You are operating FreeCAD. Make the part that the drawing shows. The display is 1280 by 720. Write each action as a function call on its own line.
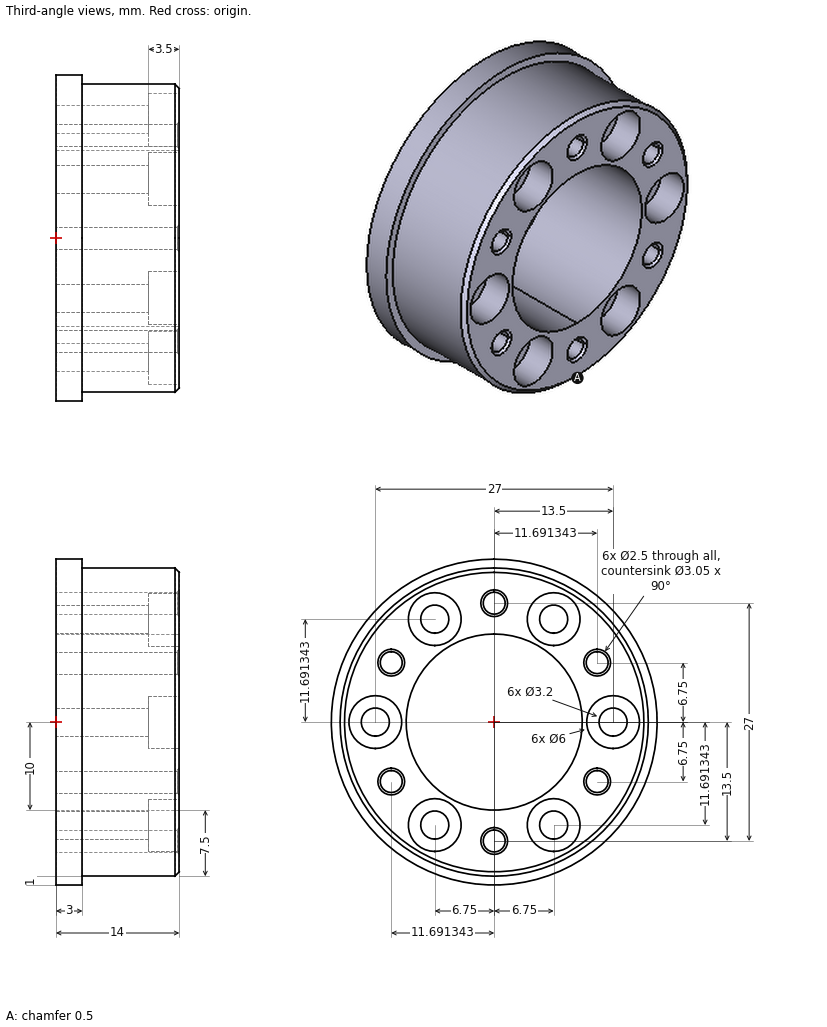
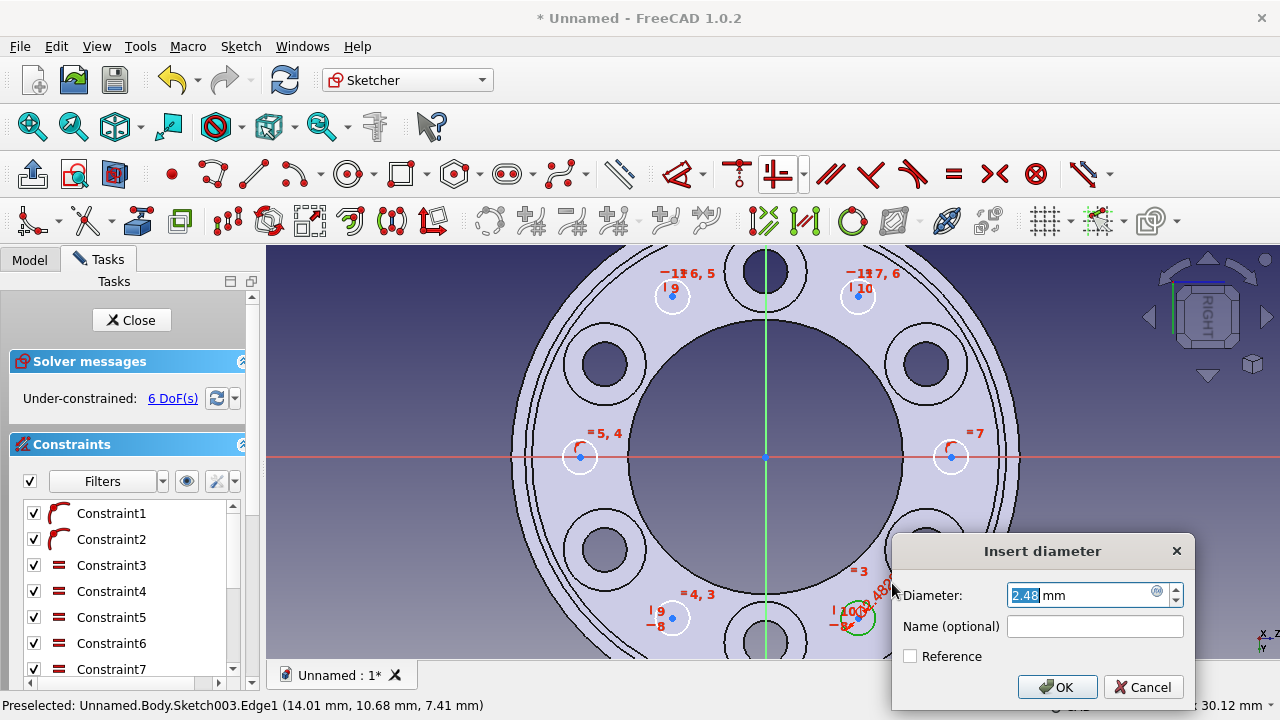
text(2.5)
key(Return)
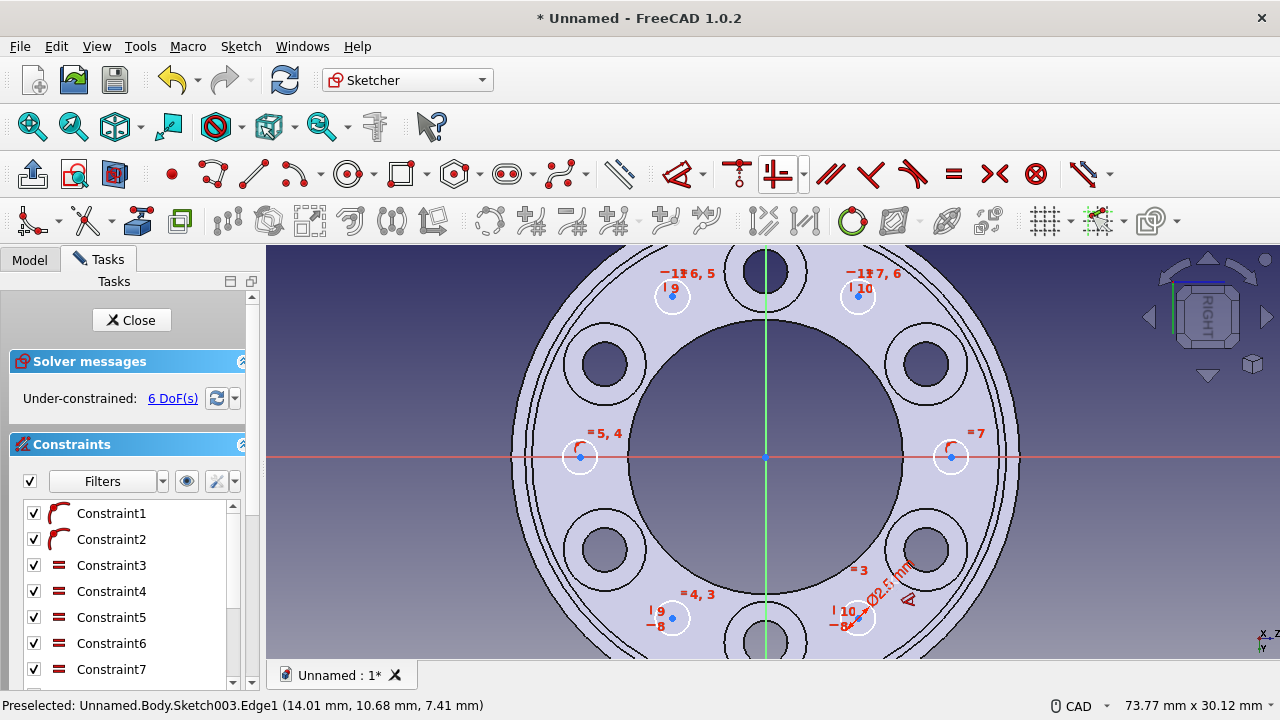
click(580, 457)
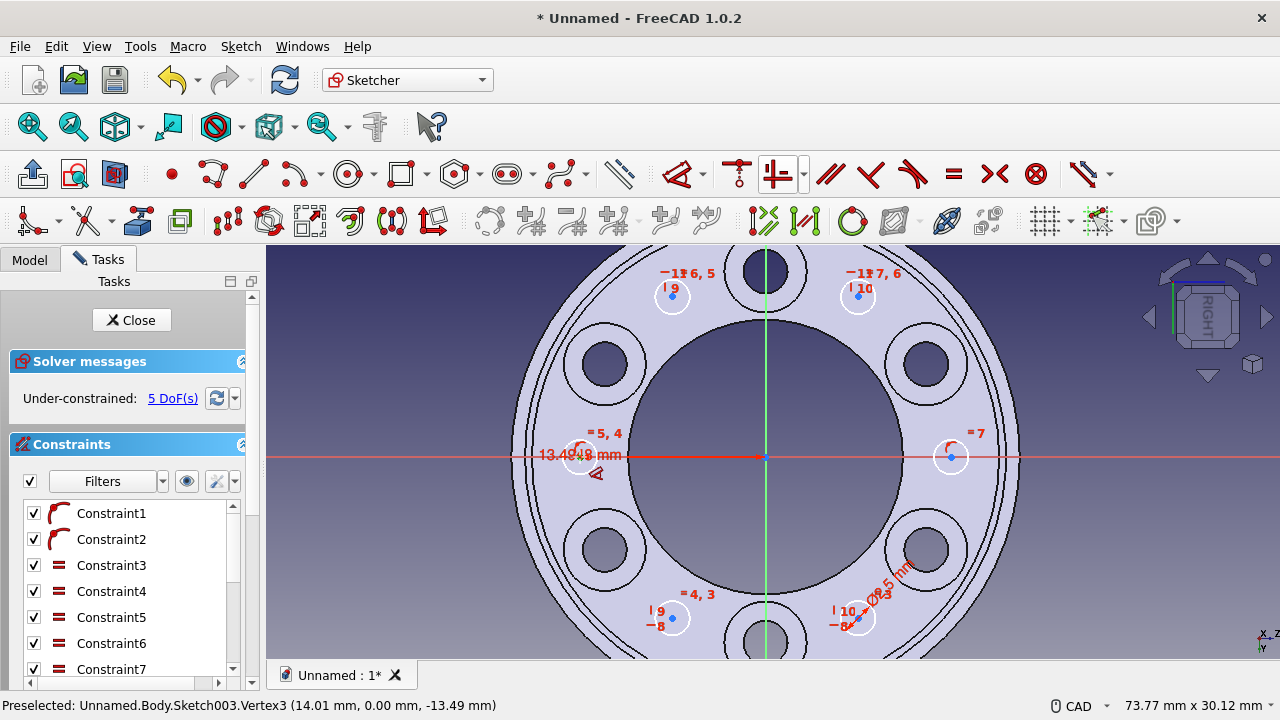
click(951, 457)
click(680, 491)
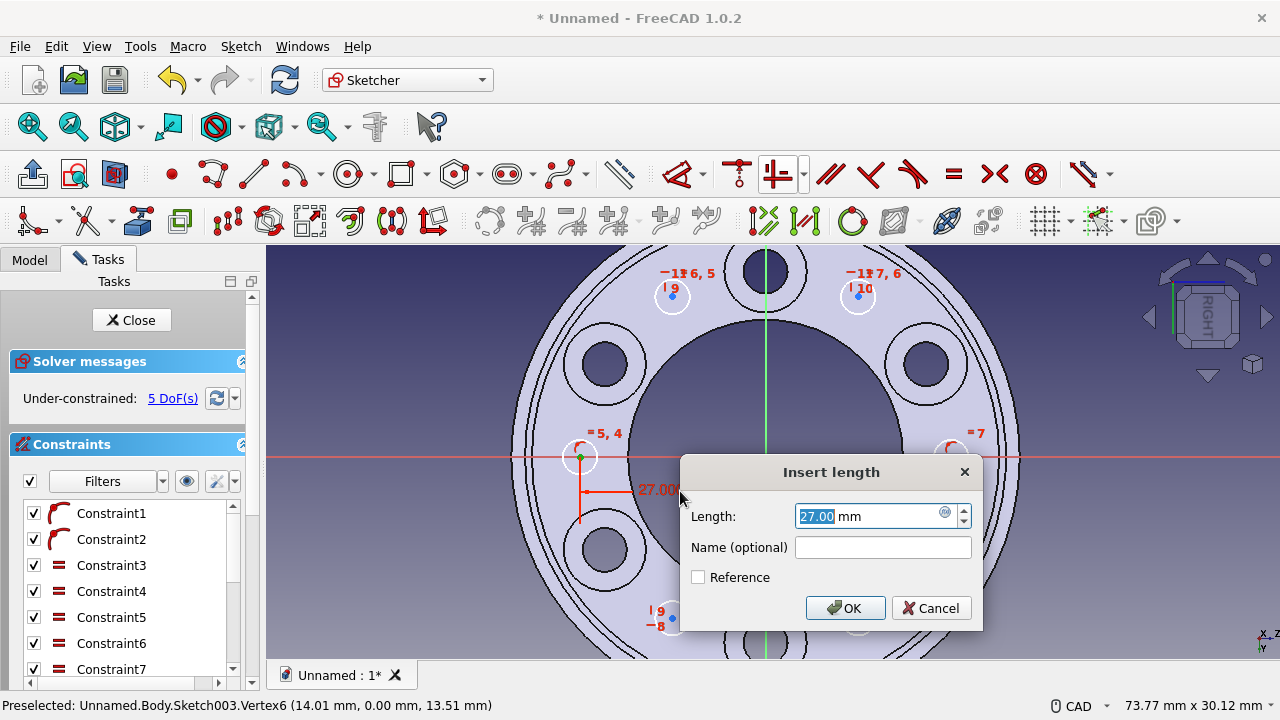
text(27)
key(Return)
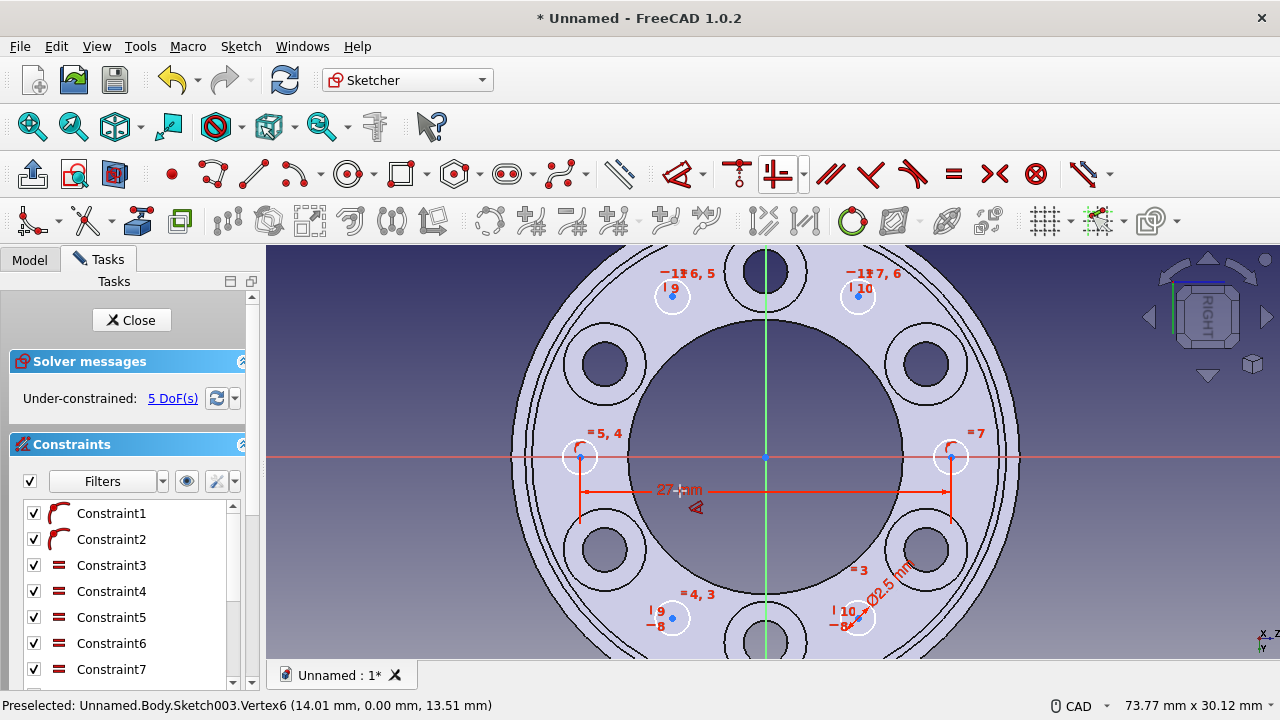
click(858, 618)
click(812, 423)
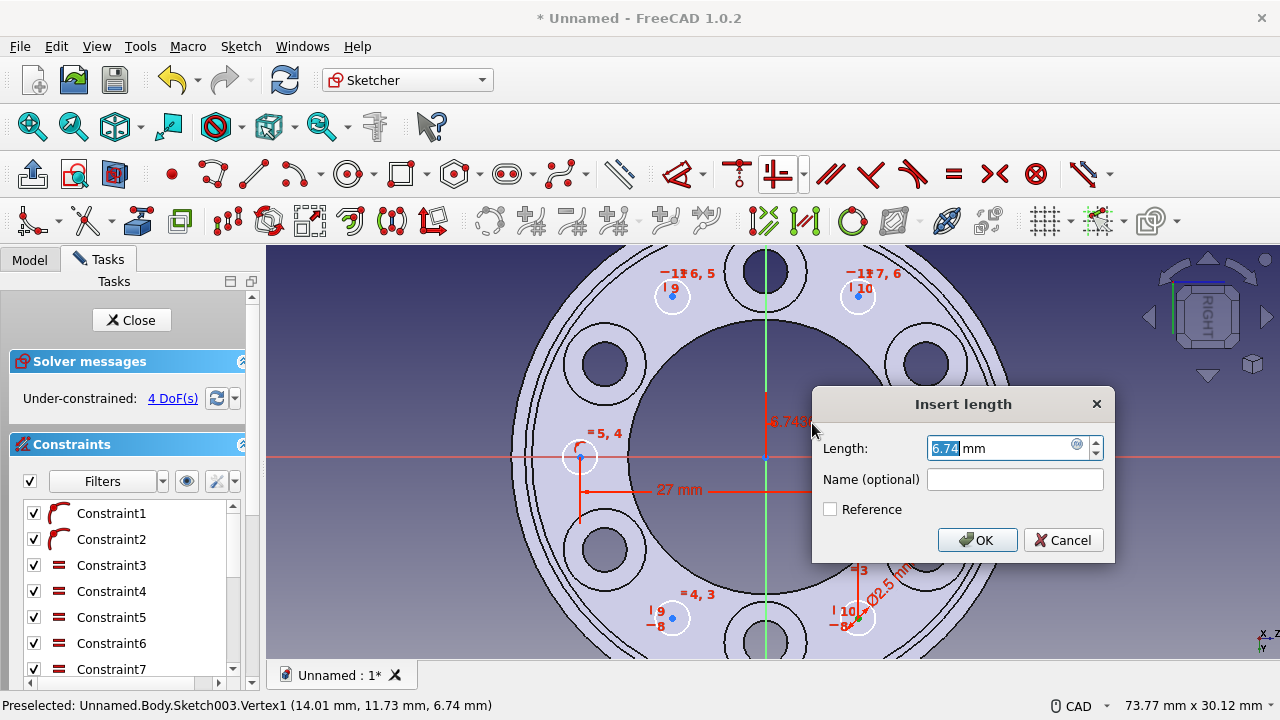
text(6.75)
key(Return)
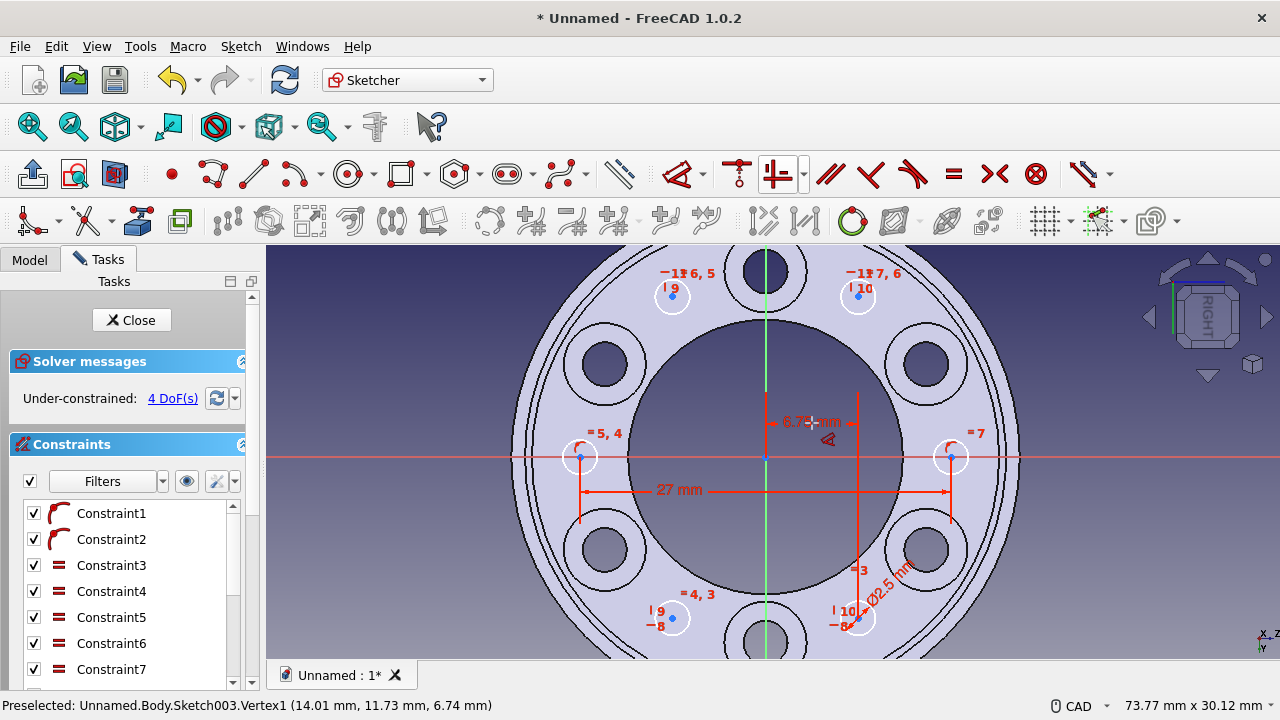
click(673, 618)
click(719, 423)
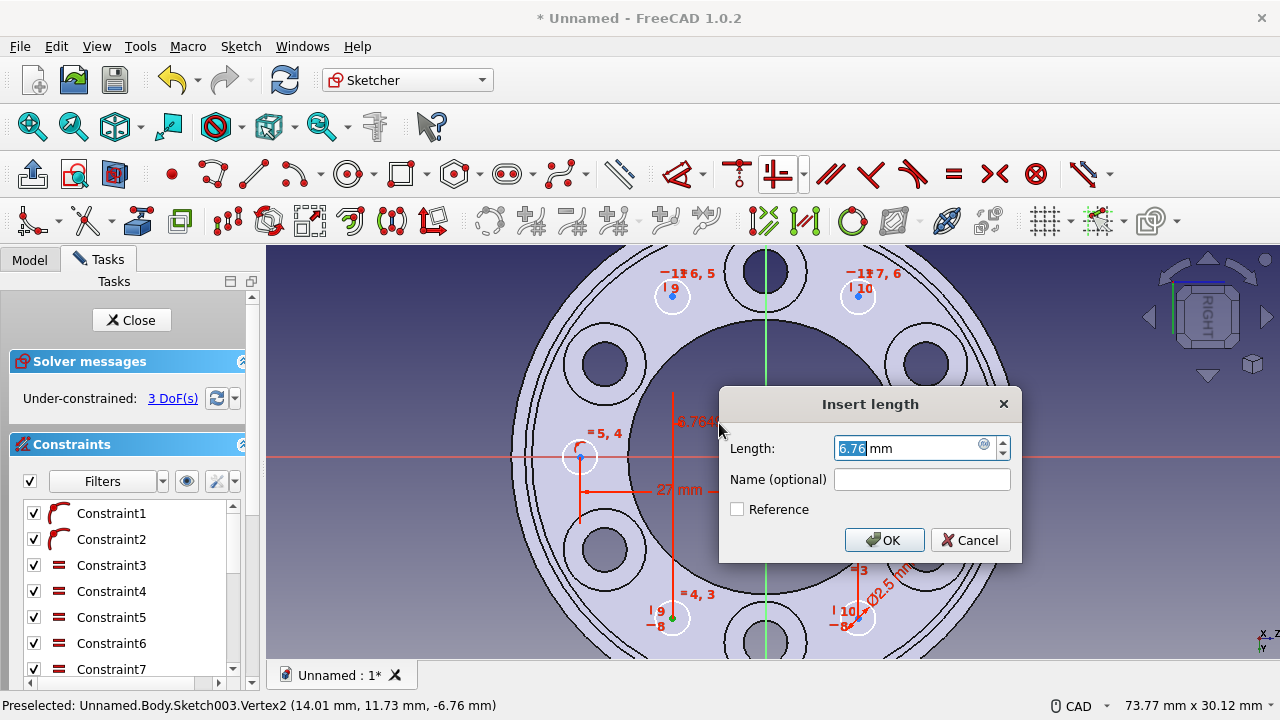
text(6.75)
key(Return)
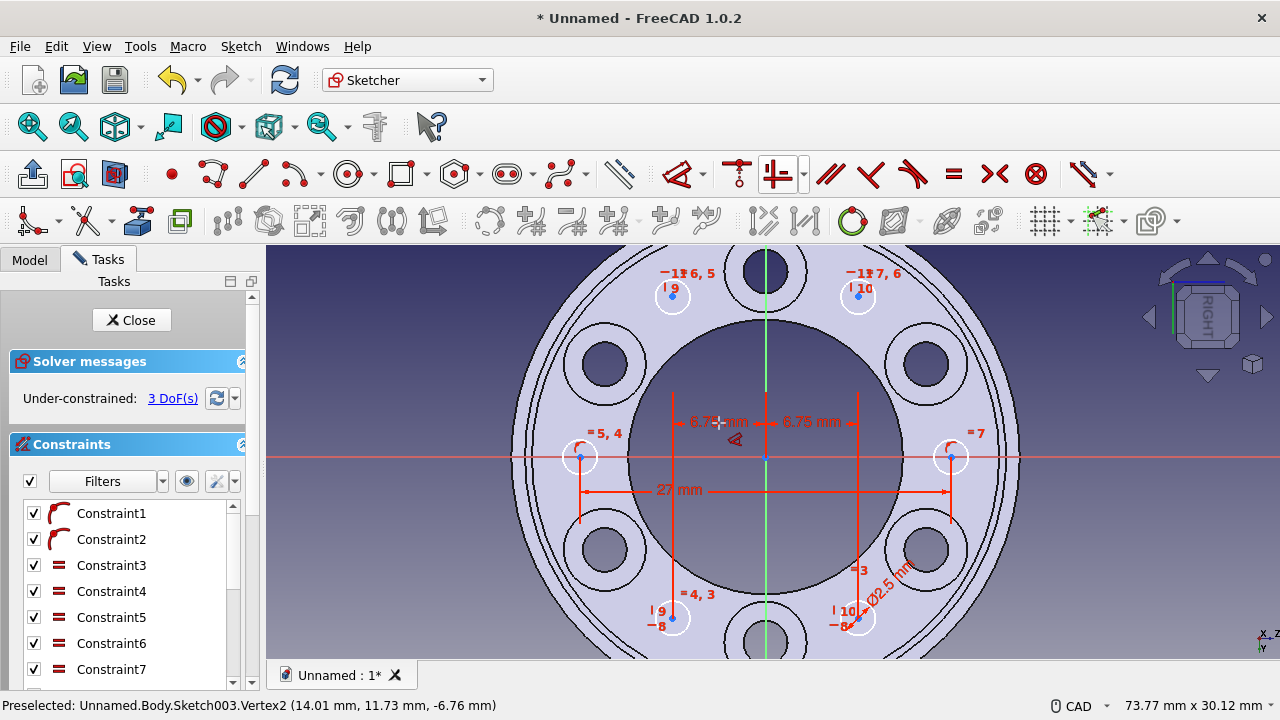
click(580, 457)
click(608, 491)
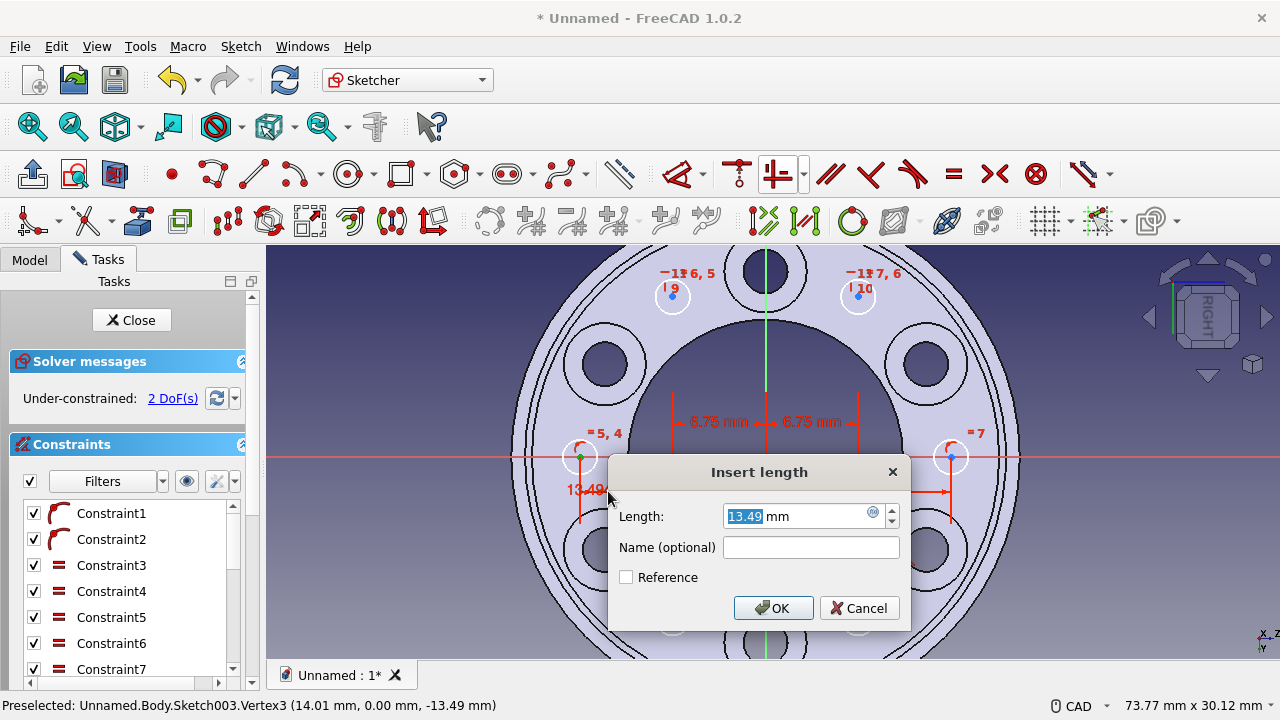
text(13.5)
key(Return)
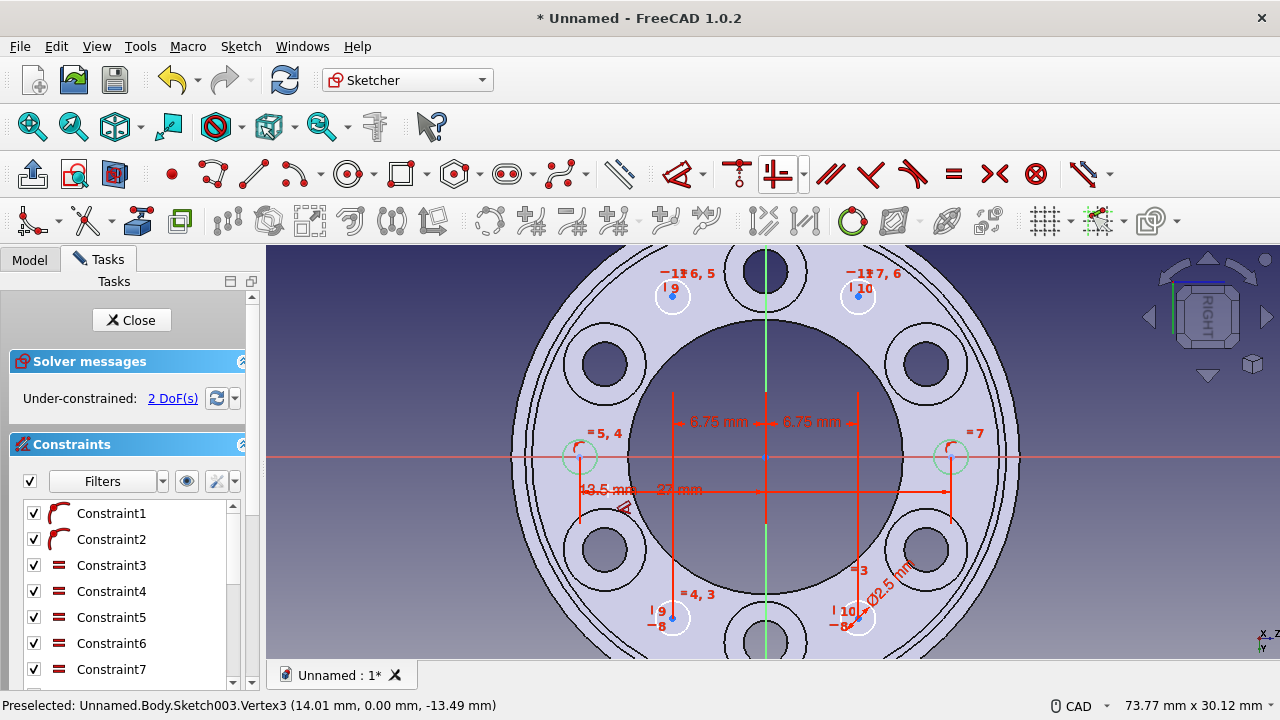
click(858, 618)
click(892, 538)